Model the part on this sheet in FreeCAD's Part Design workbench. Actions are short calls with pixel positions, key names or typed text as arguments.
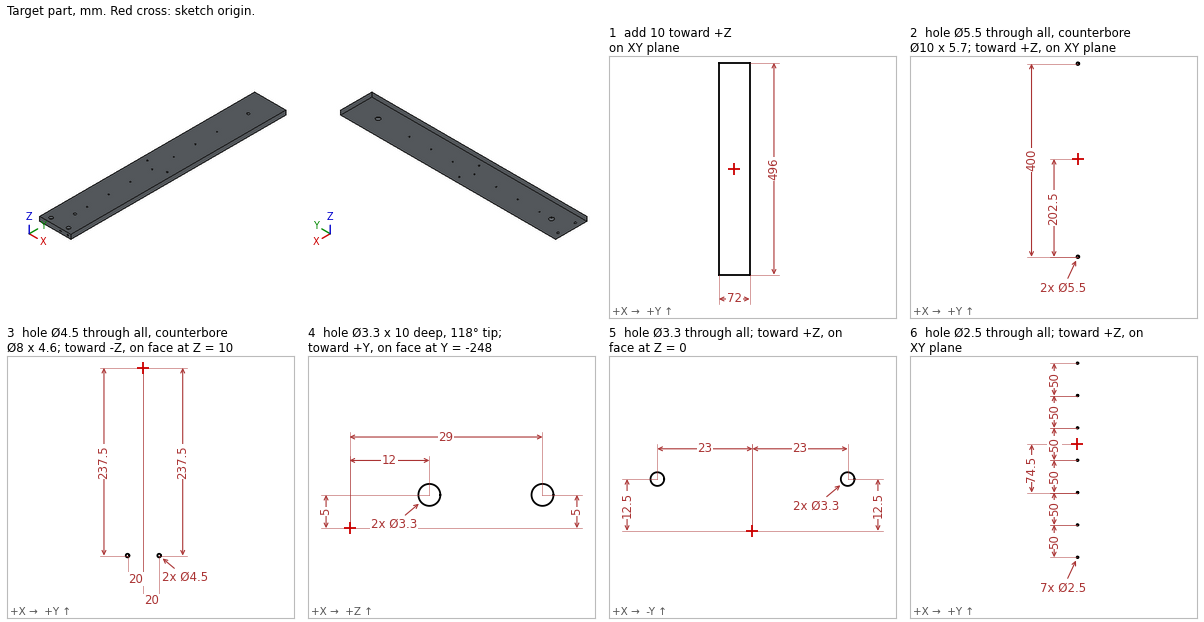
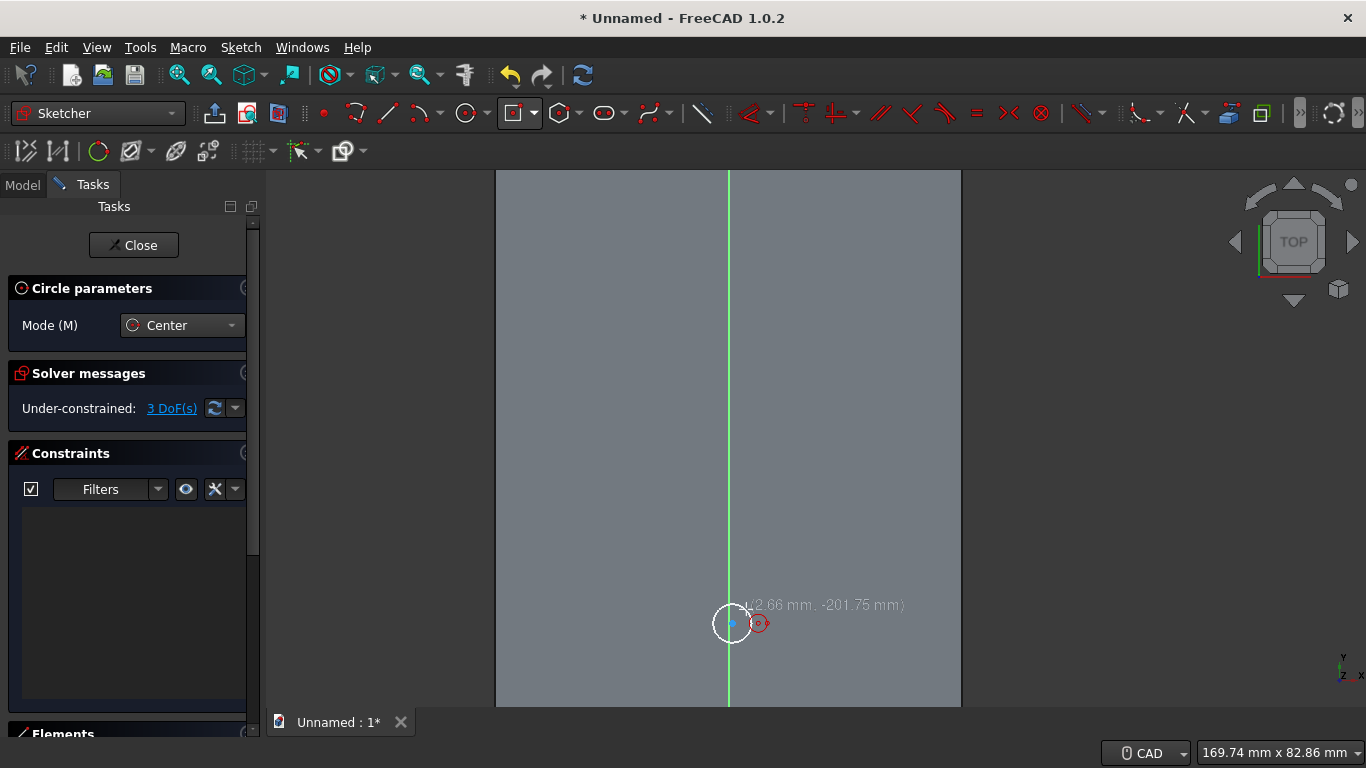
scroll(750, 614, down, 10)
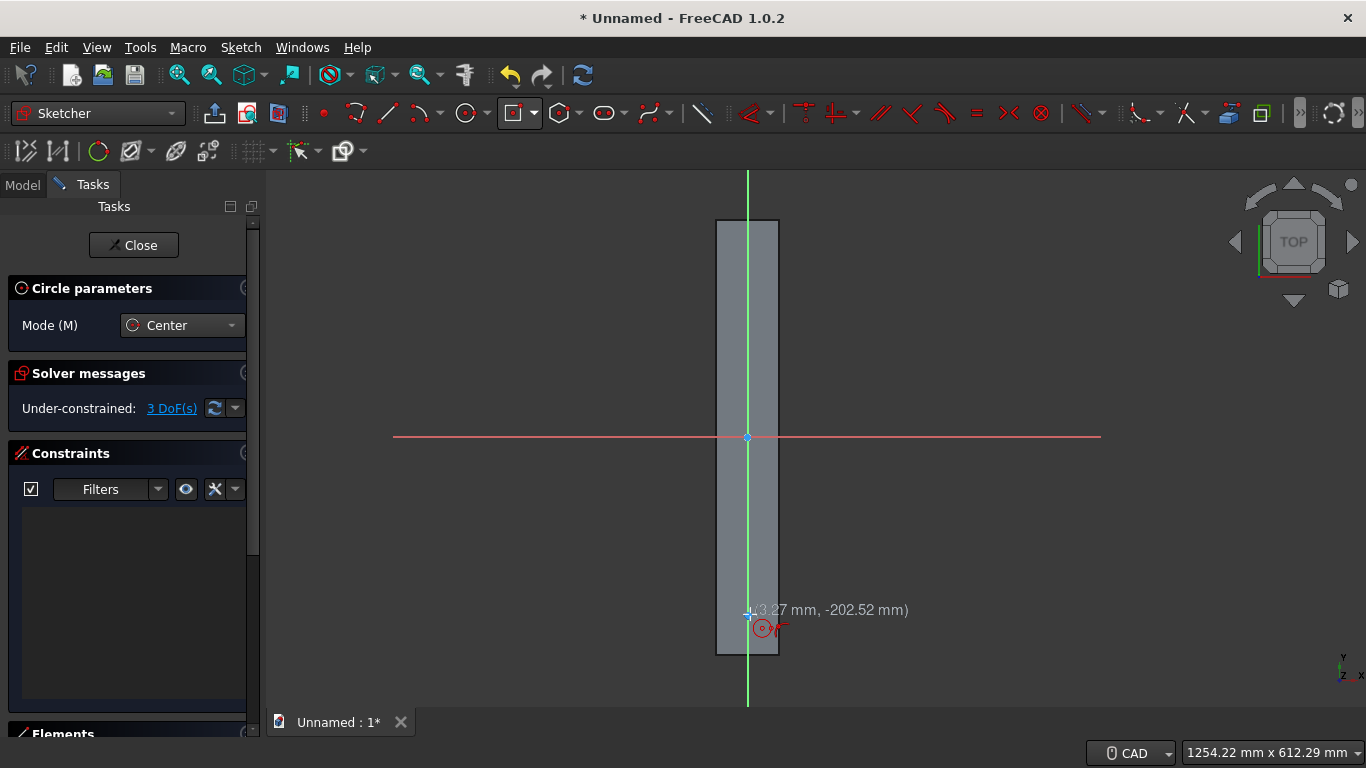
scroll(748, 264, up, 12)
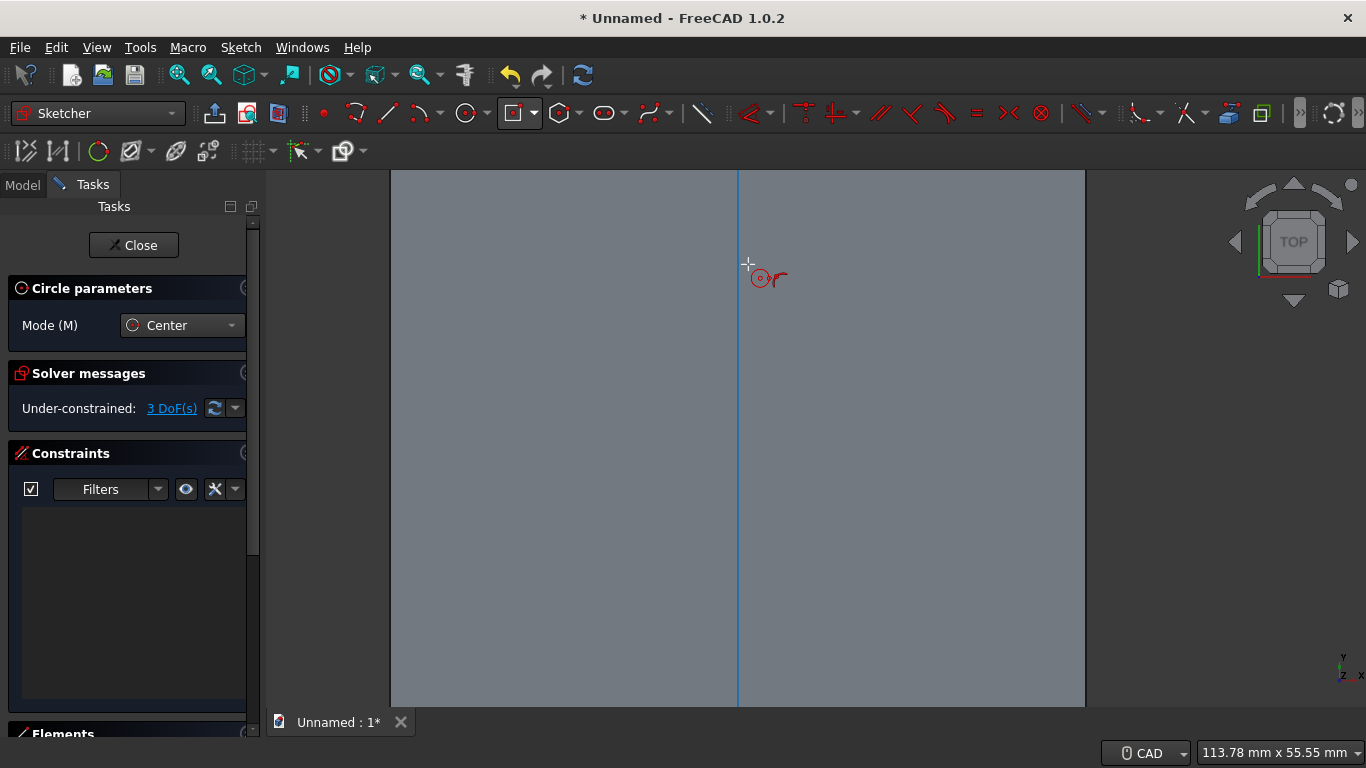
scroll(748, 263, down, 12)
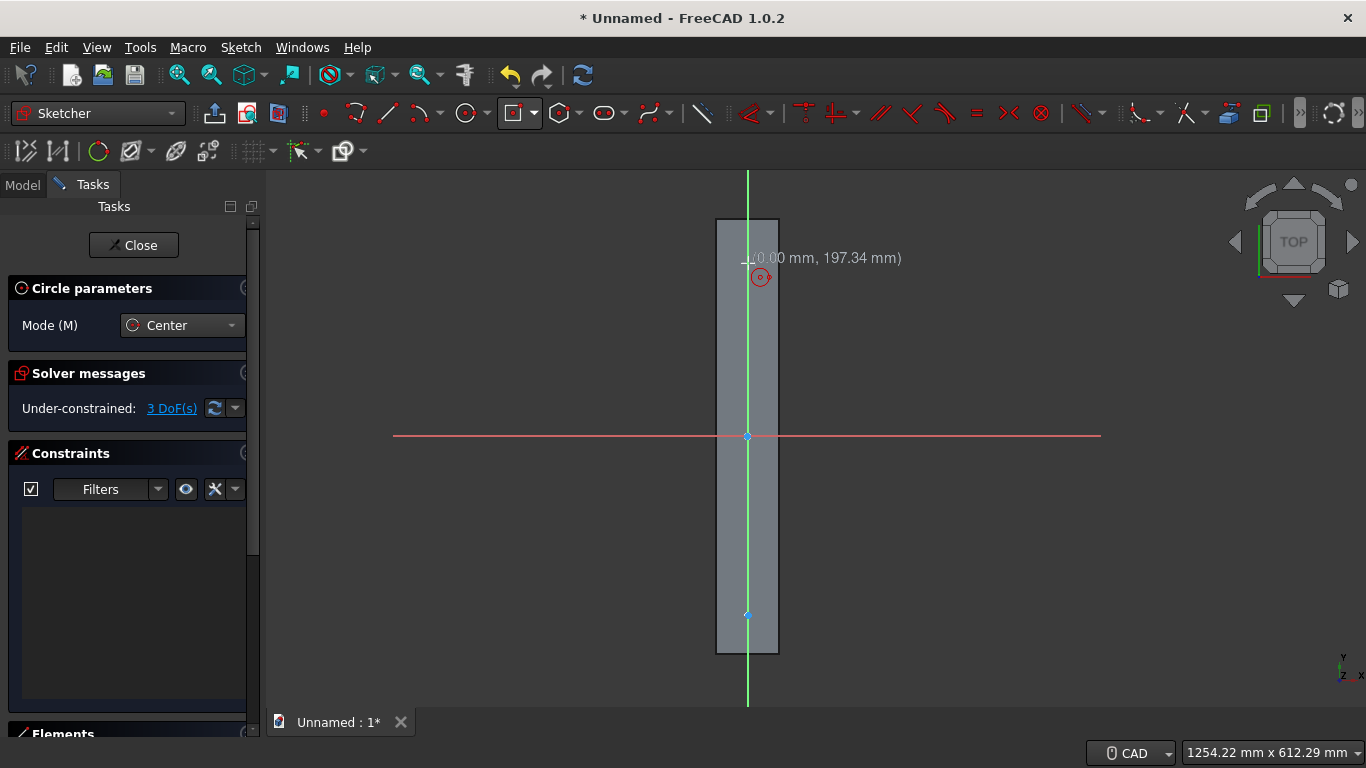
click(748, 263)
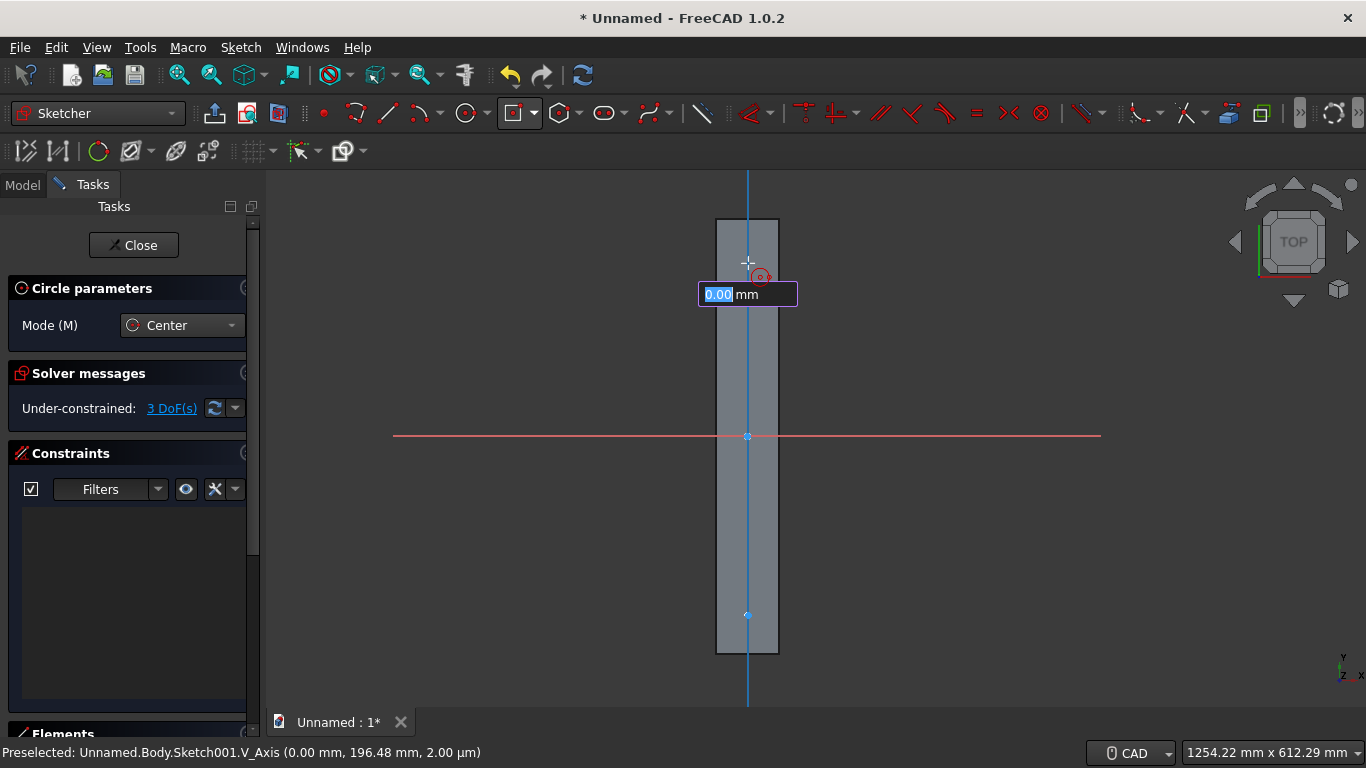
scroll(750, 262, up, 10)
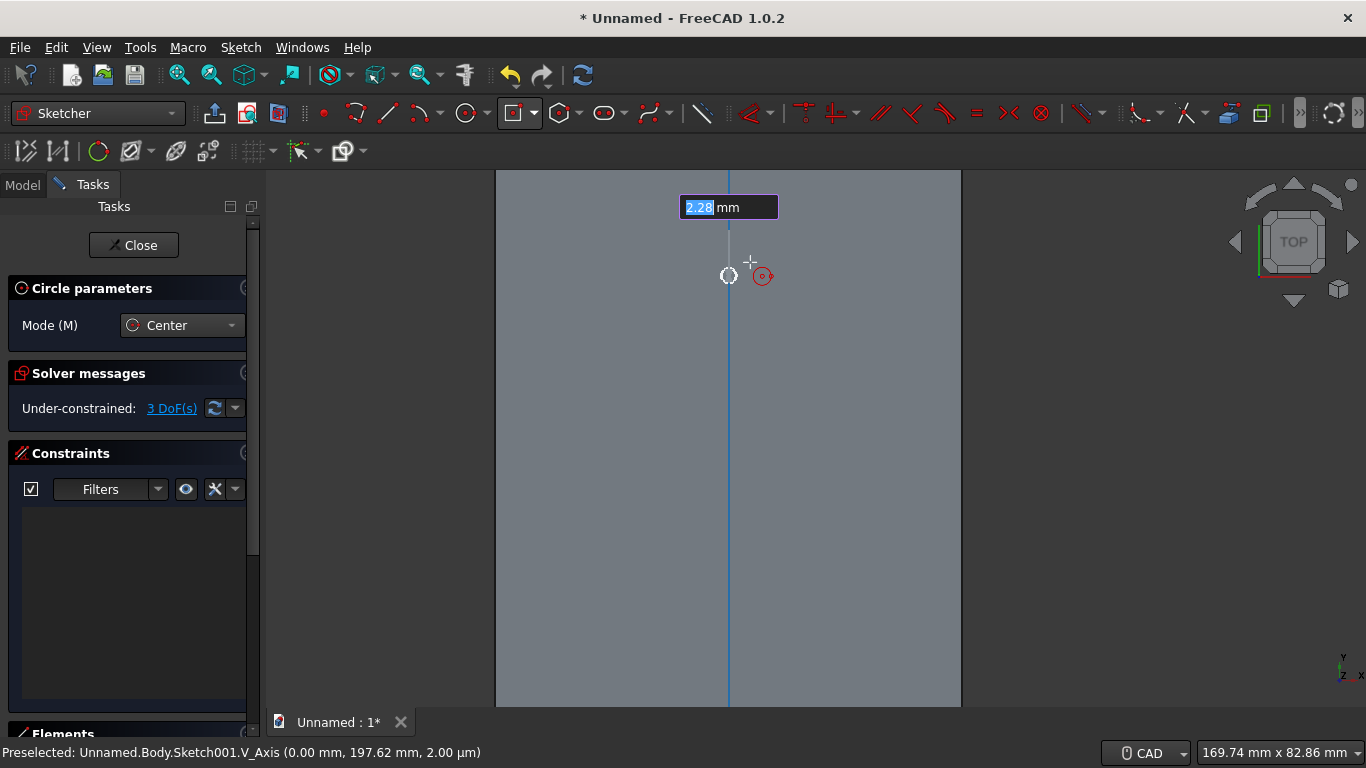
click(746, 263)
key(Escape)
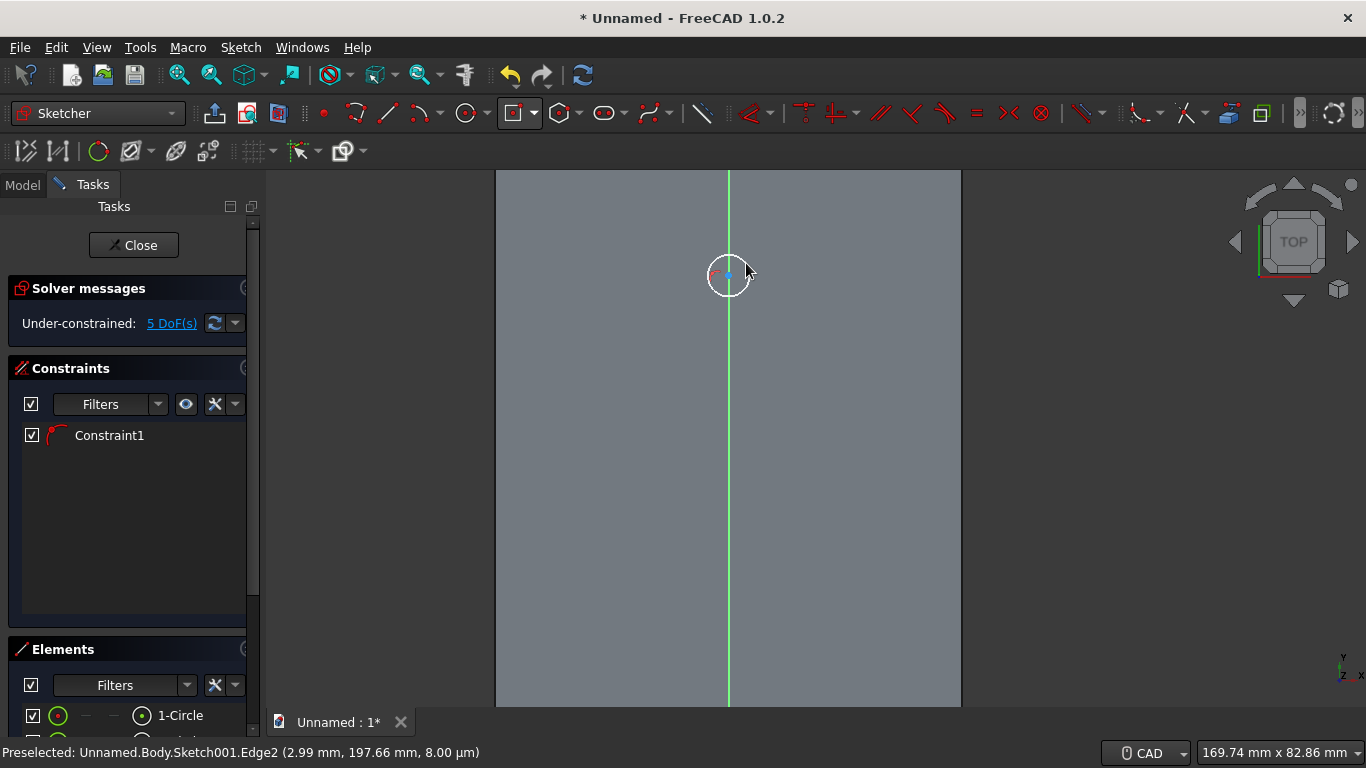
scroll(750, 262, down, 10)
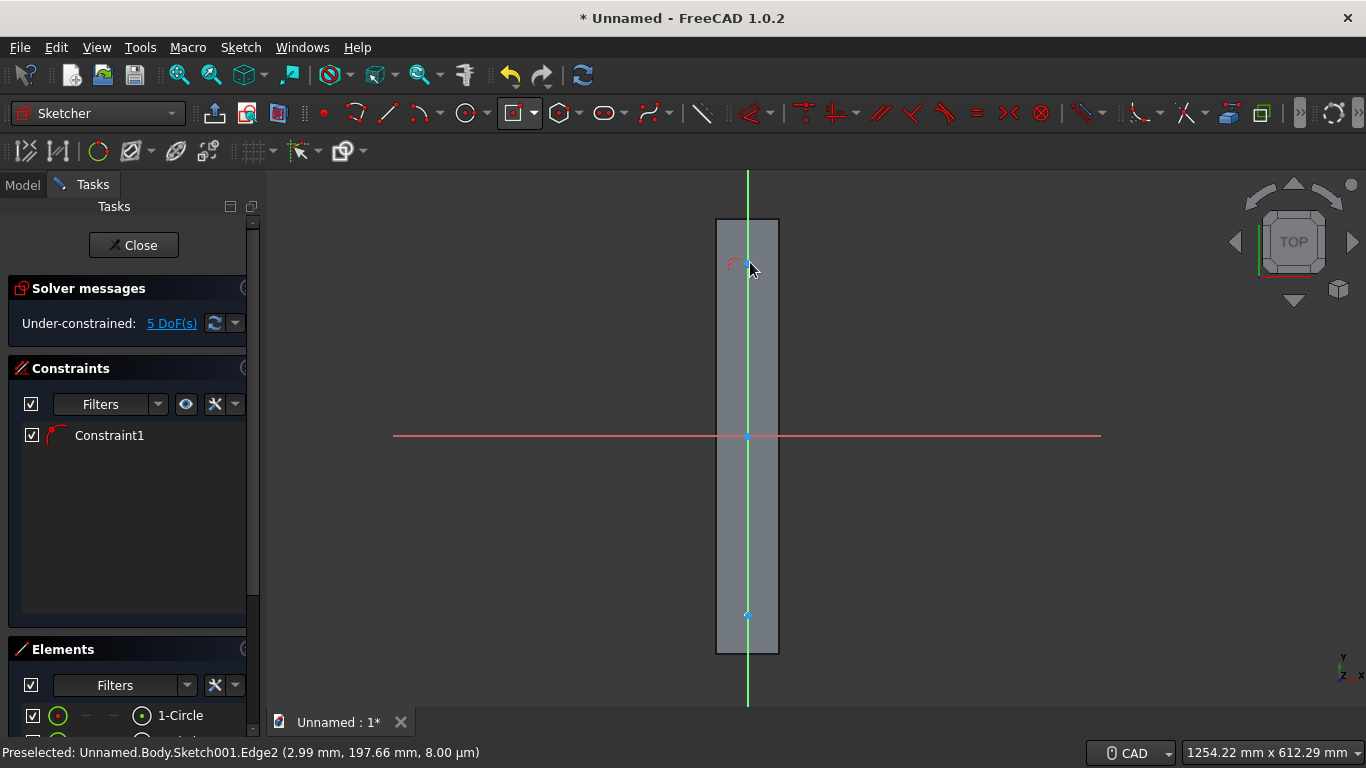
scroll(750, 613, up, 9)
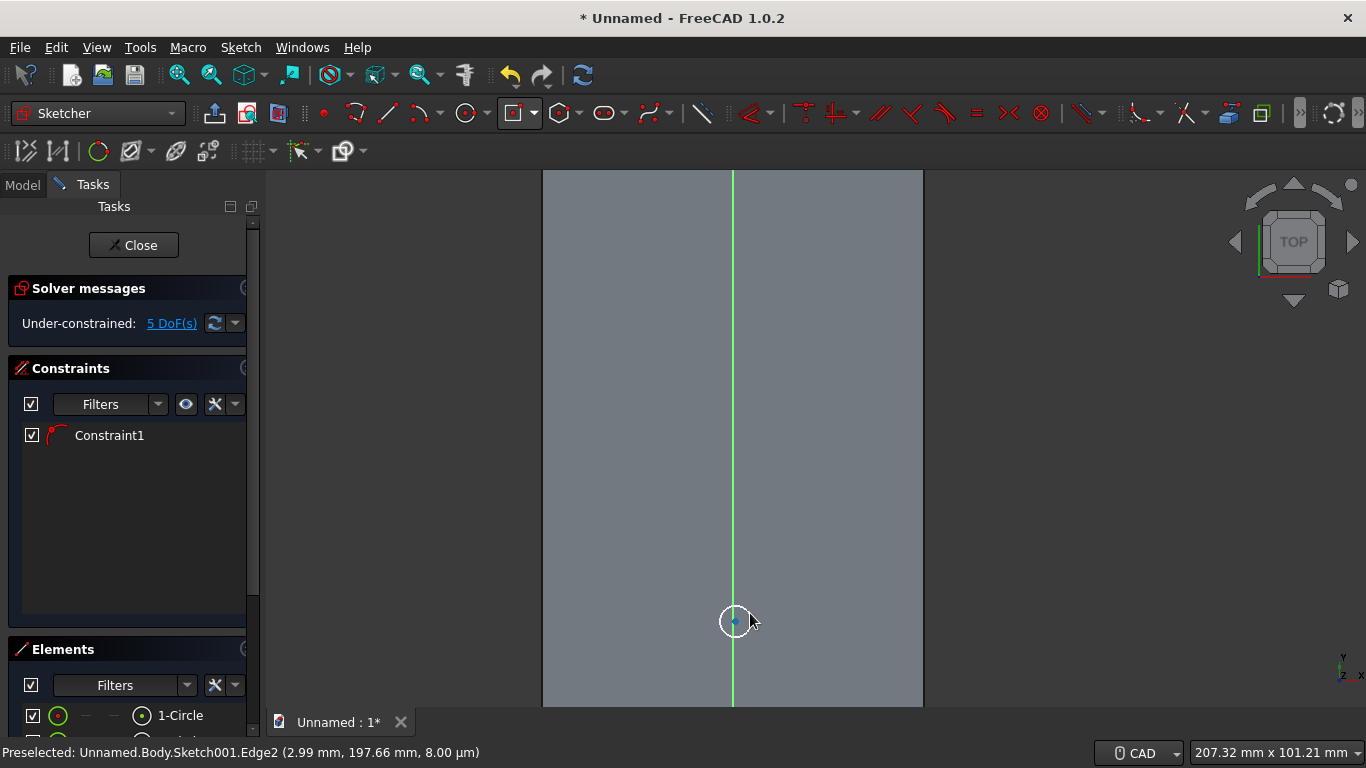
click(747, 610)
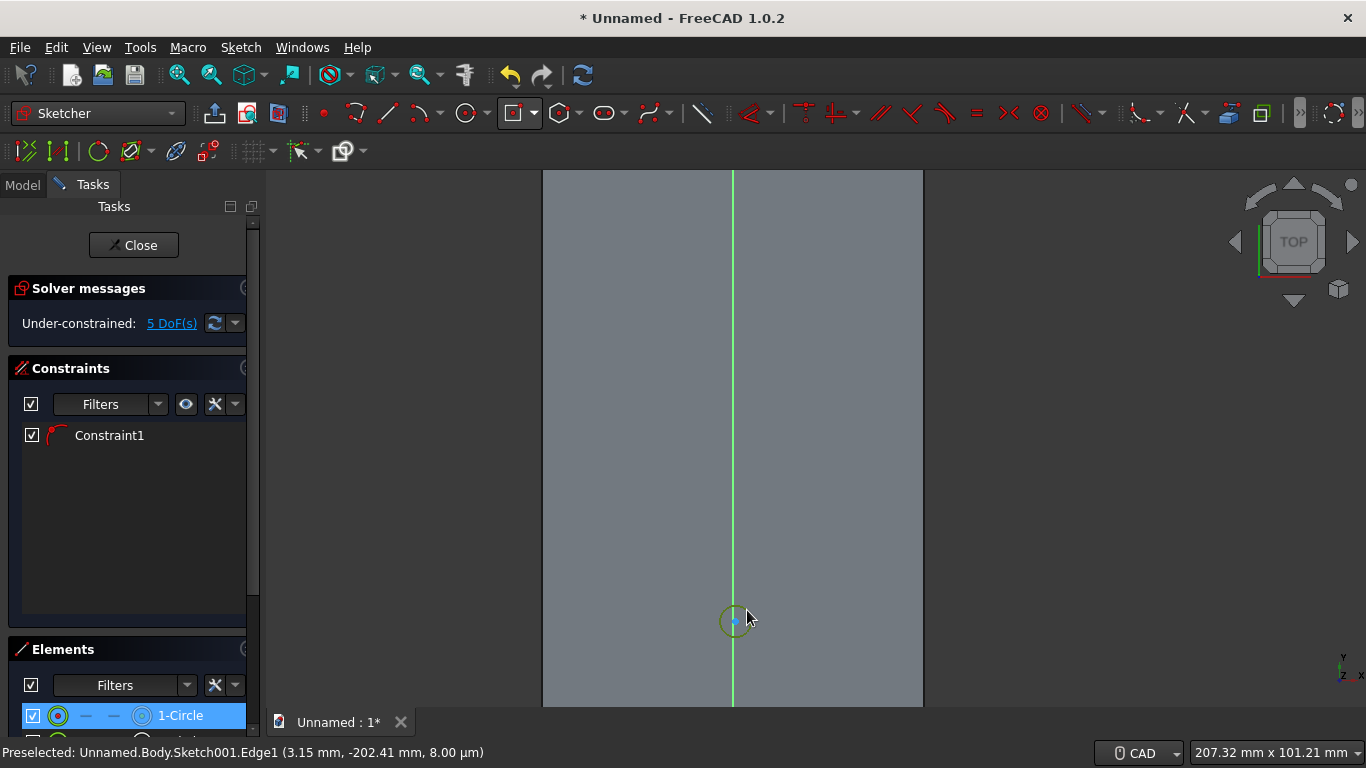
scroll(750, 614, down, 9)